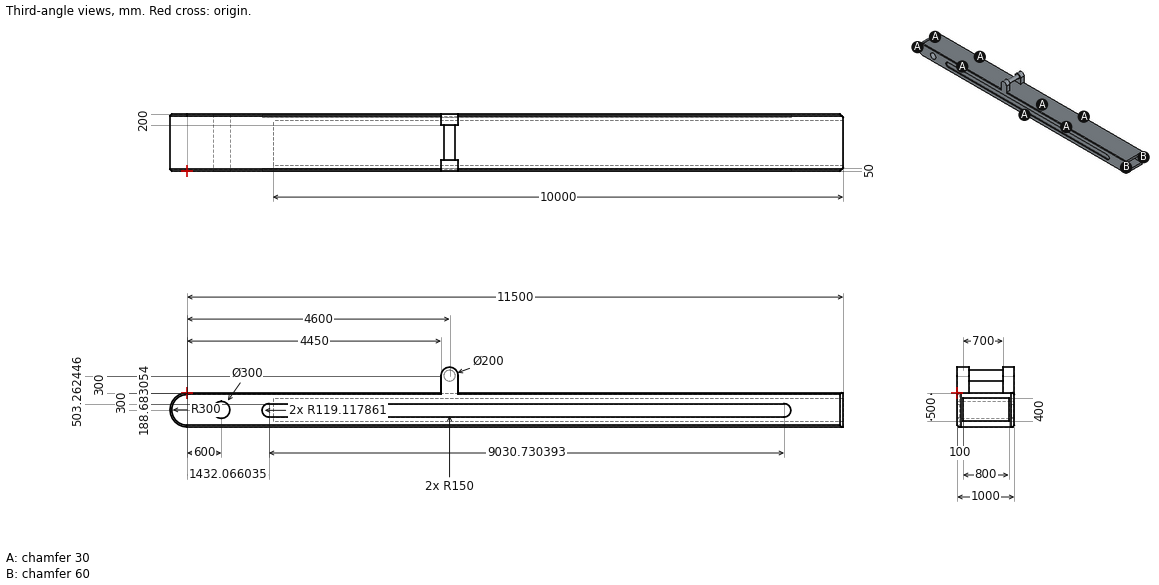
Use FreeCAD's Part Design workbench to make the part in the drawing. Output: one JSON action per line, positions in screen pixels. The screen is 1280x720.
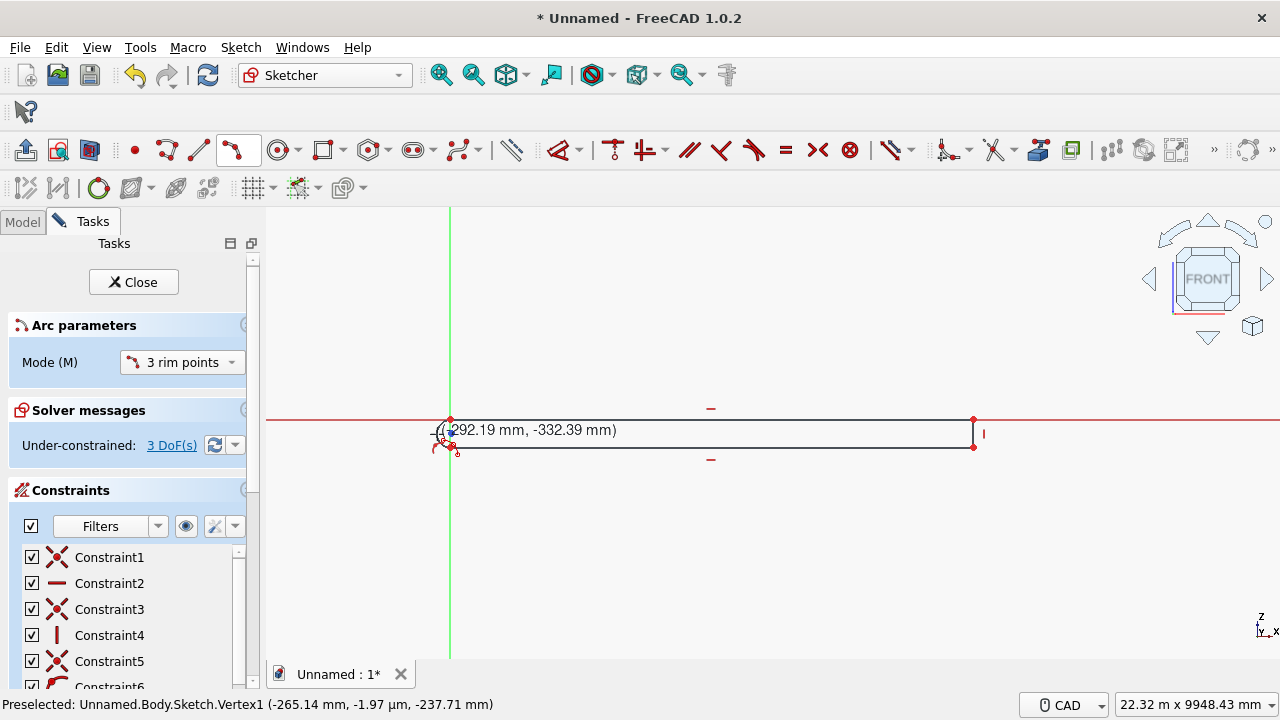
{"action": "left_click", "coordinate": [278, 150]}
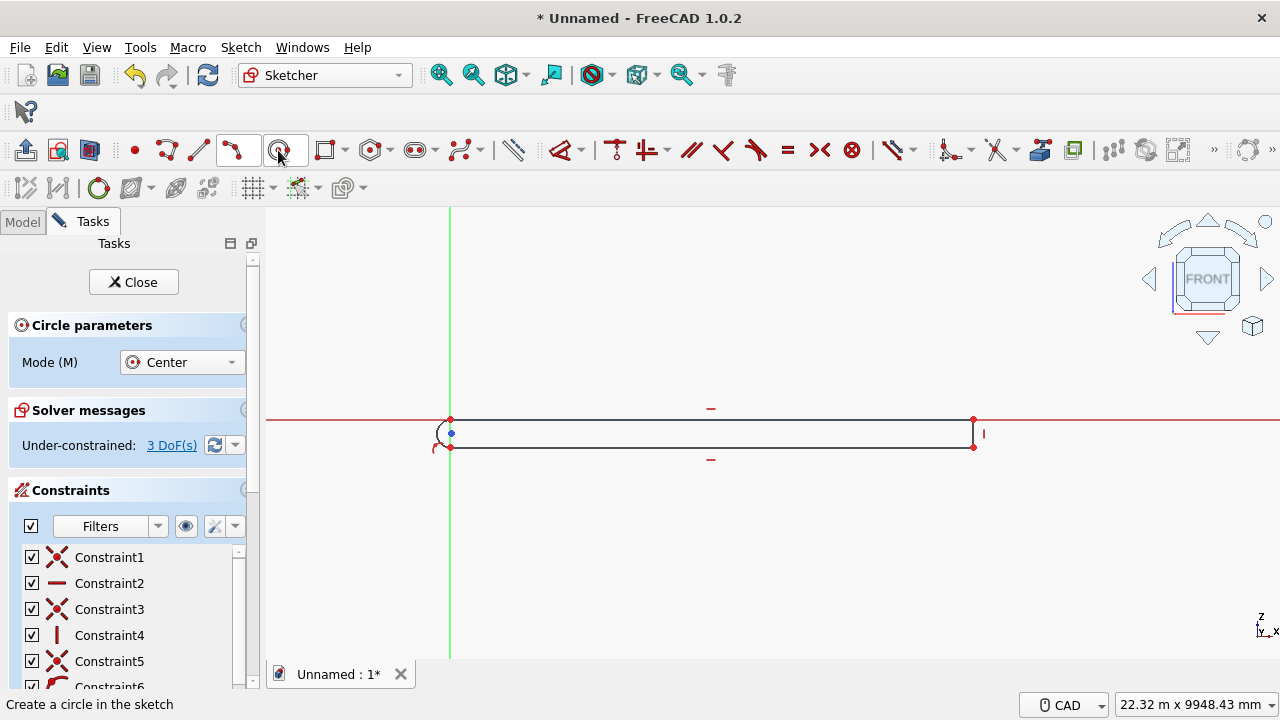
{"action": "scroll", "coordinate": [478, 434], "scroll_direction": "up", "scroll_amount": 7}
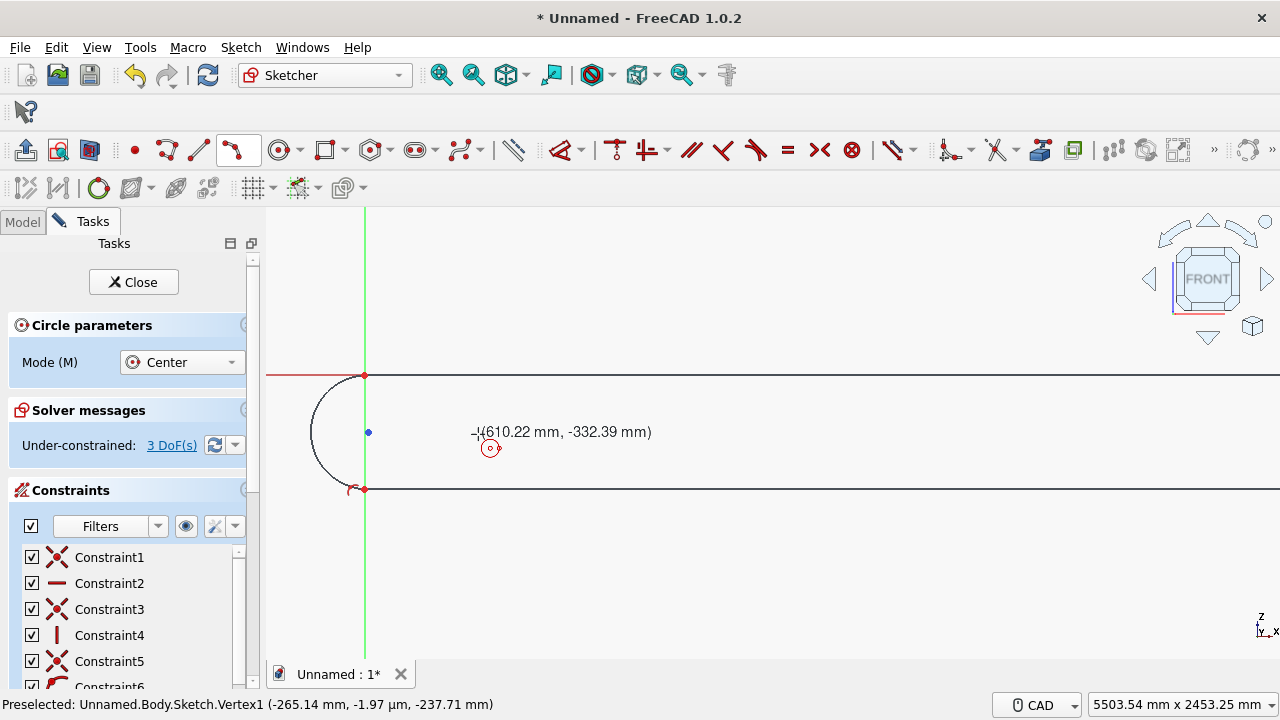
{"action": "scroll", "coordinate": [478, 434], "scroll_direction": "down", "scroll_amount": 7}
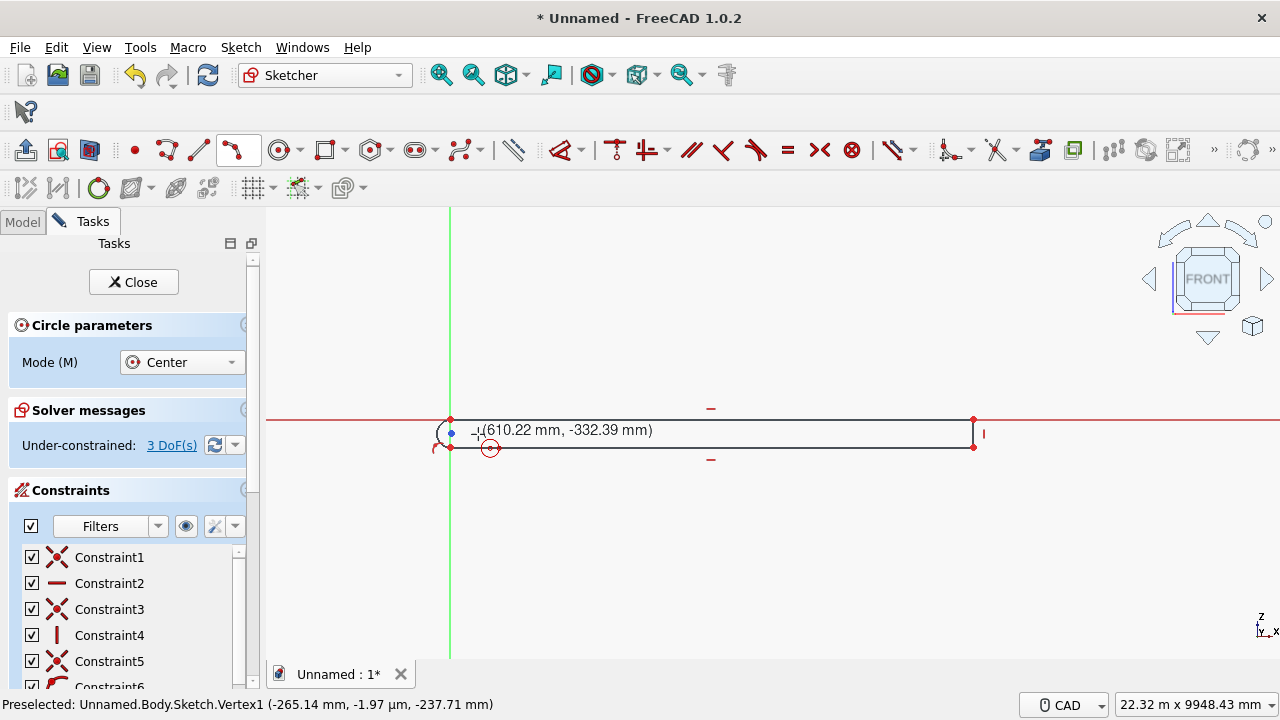
{"action": "left_click", "coordinate": [478, 434]}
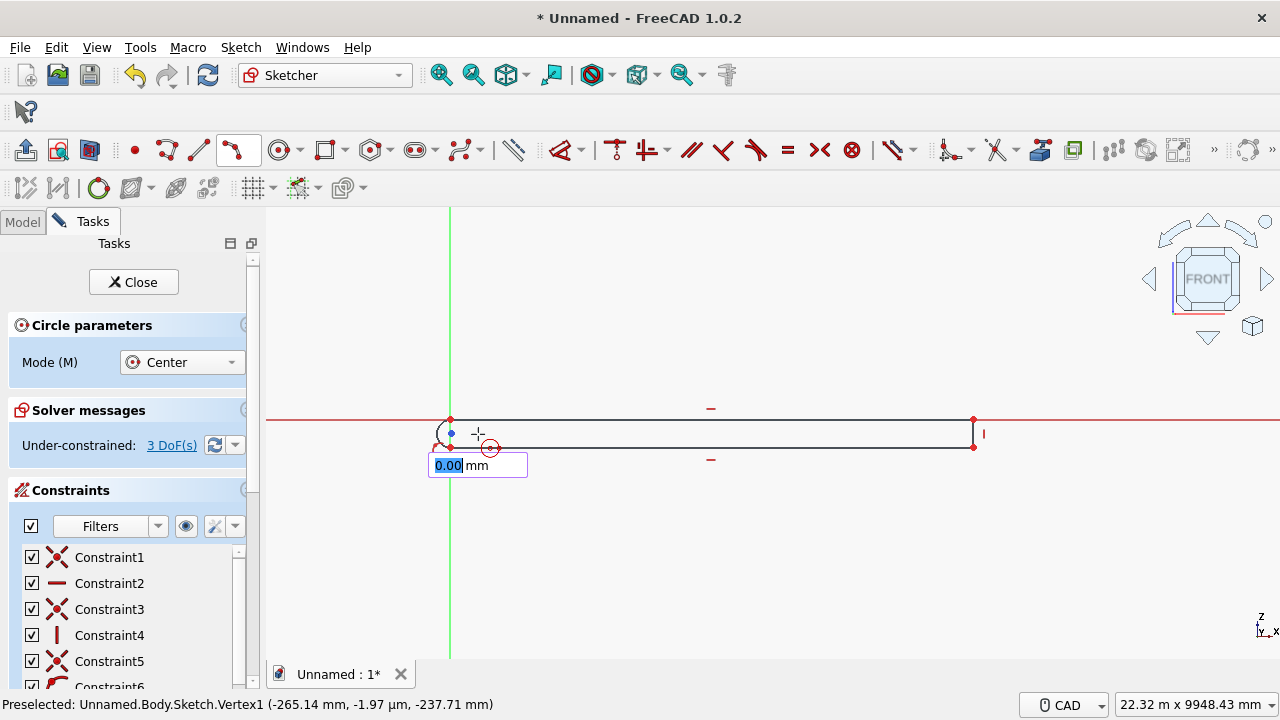
{"action": "scroll", "coordinate": [484, 431], "scroll_direction": "up", "scroll_amount": 5}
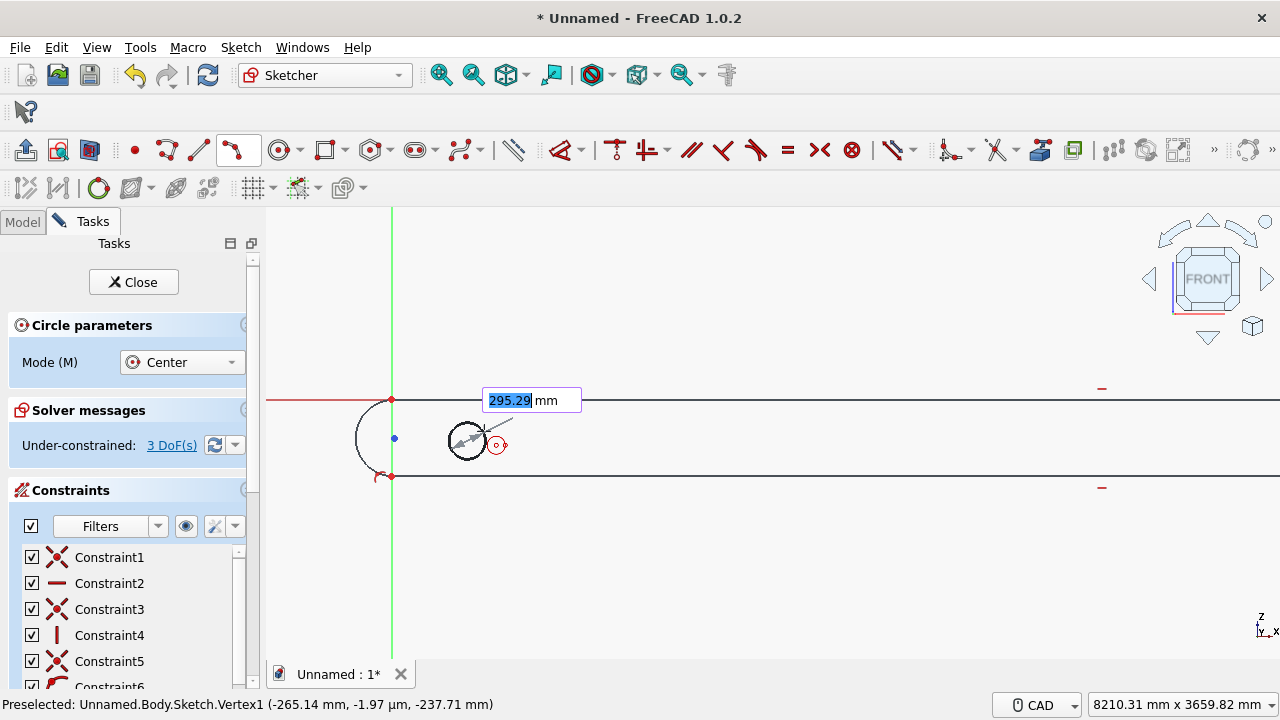
{"action": "left_click", "coordinate": [483, 431]}
{"action": "key", "text": "Escape"}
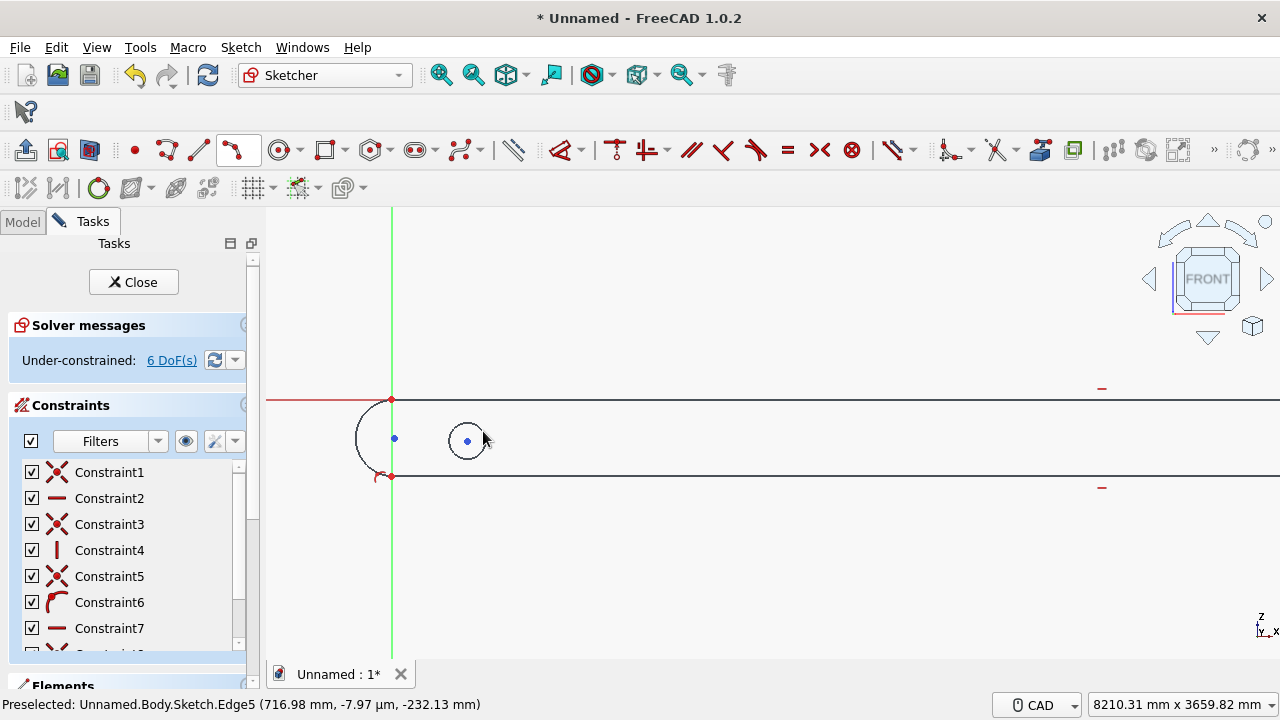
{"action": "left_click", "coordinate": [394, 438]}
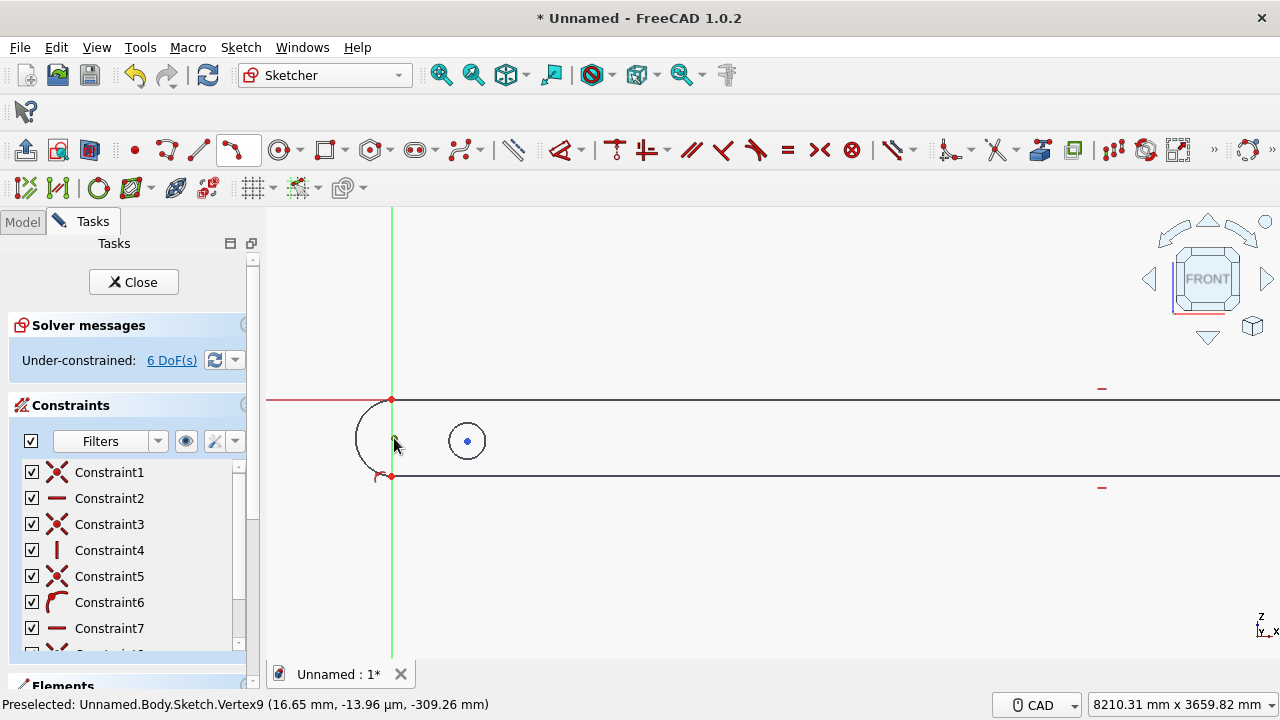
{"action": "left_click", "coordinate": [392, 603]}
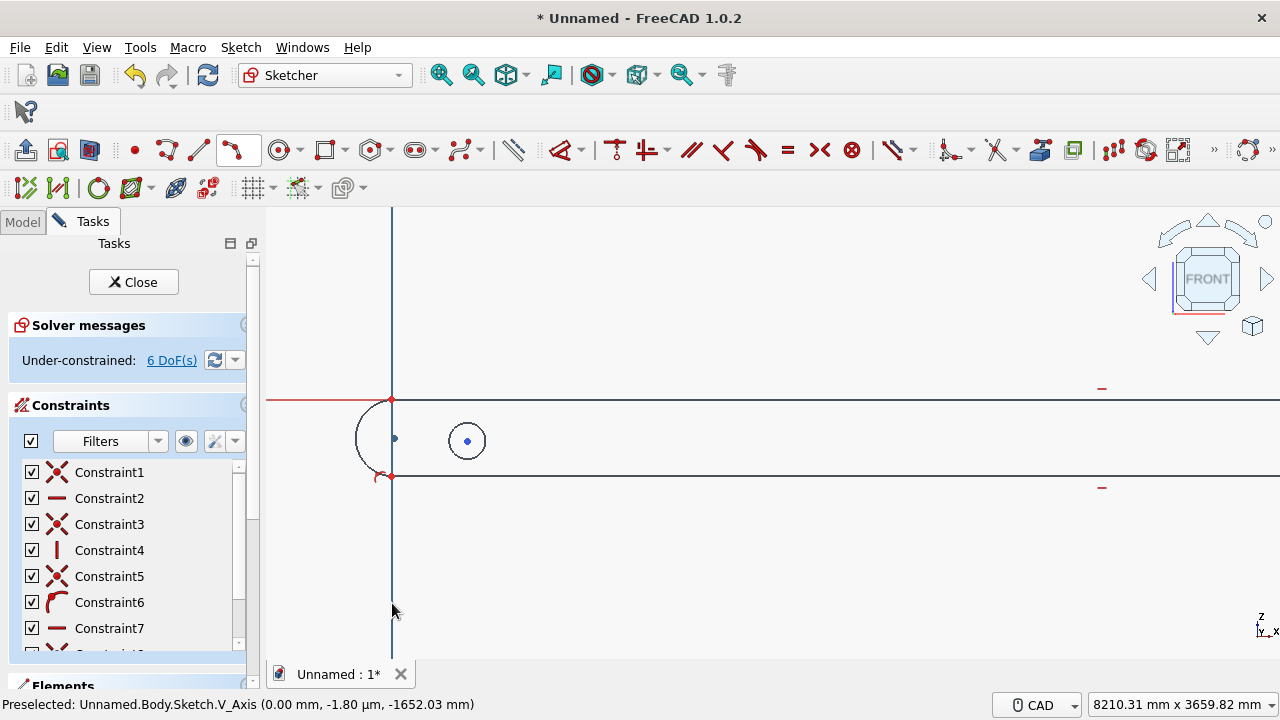
{"action": "left_click", "coordinate": [616, 150]}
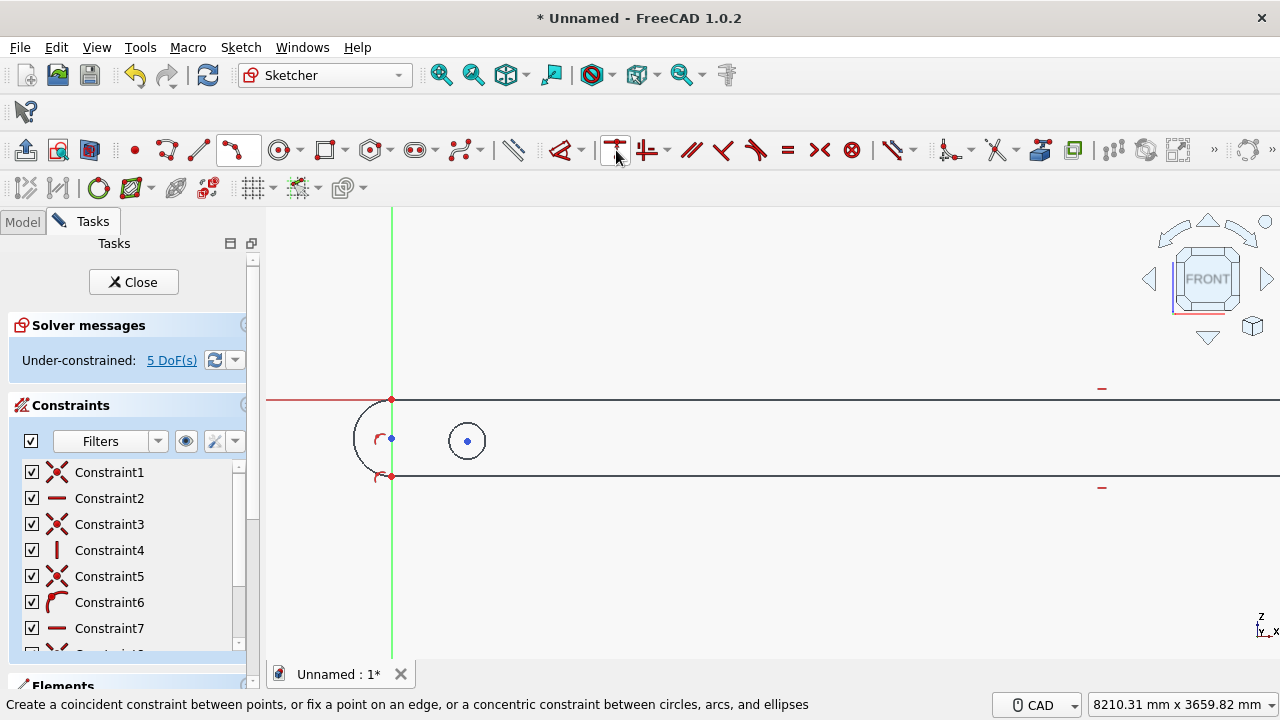
{"action": "left_click", "coordinate": [361, 416]}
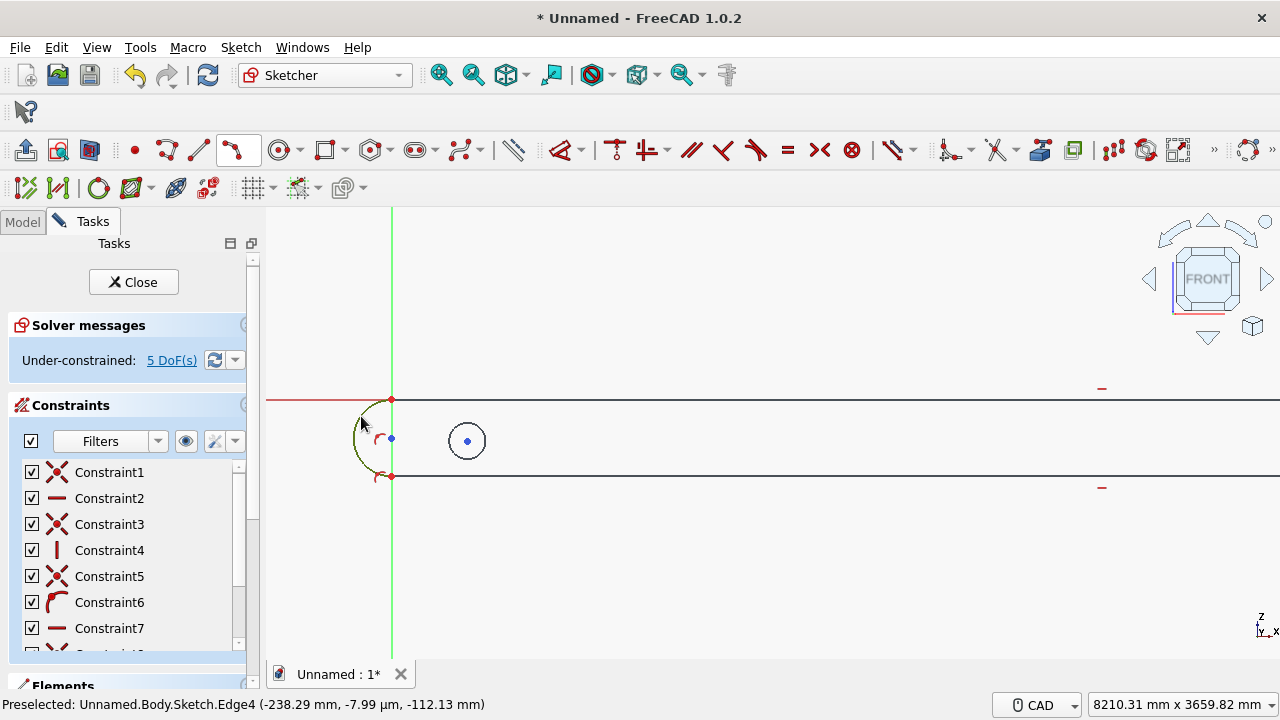
{"action": "left_click", "coordinate": [584, 150]}